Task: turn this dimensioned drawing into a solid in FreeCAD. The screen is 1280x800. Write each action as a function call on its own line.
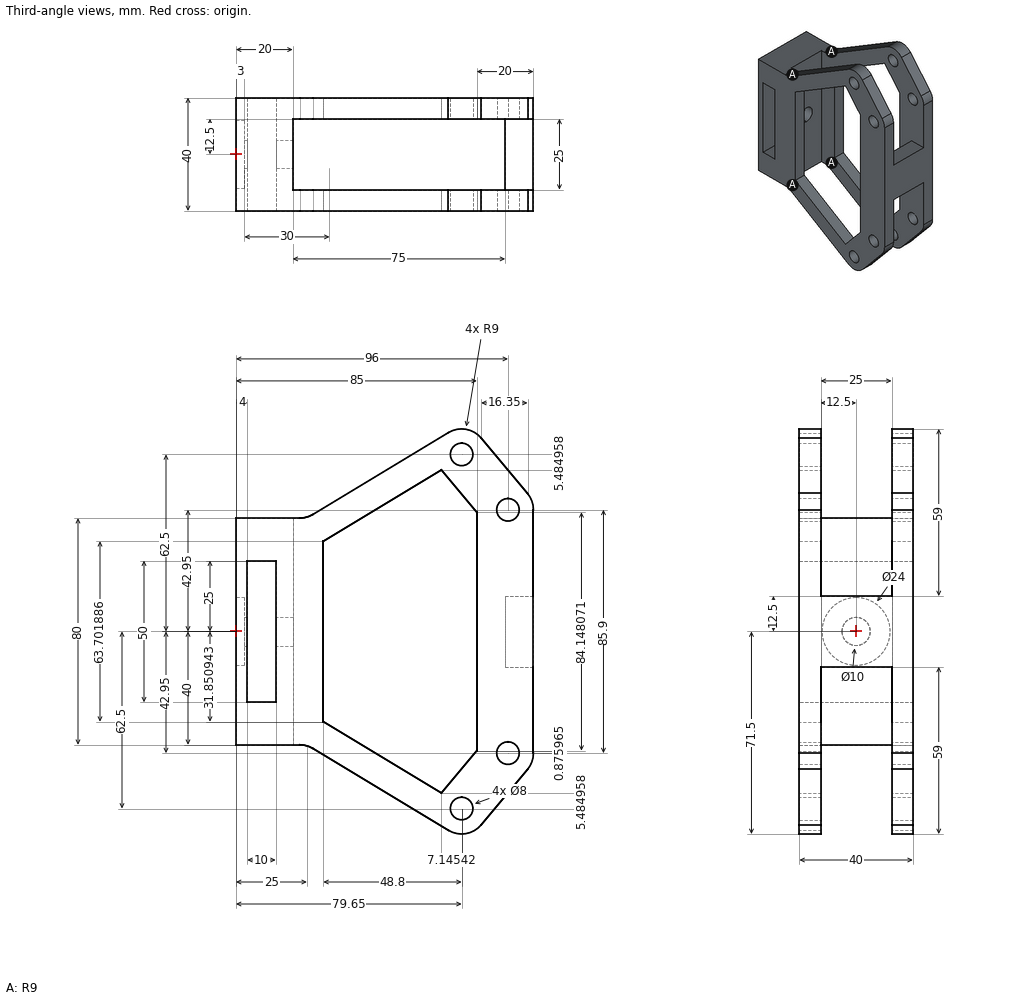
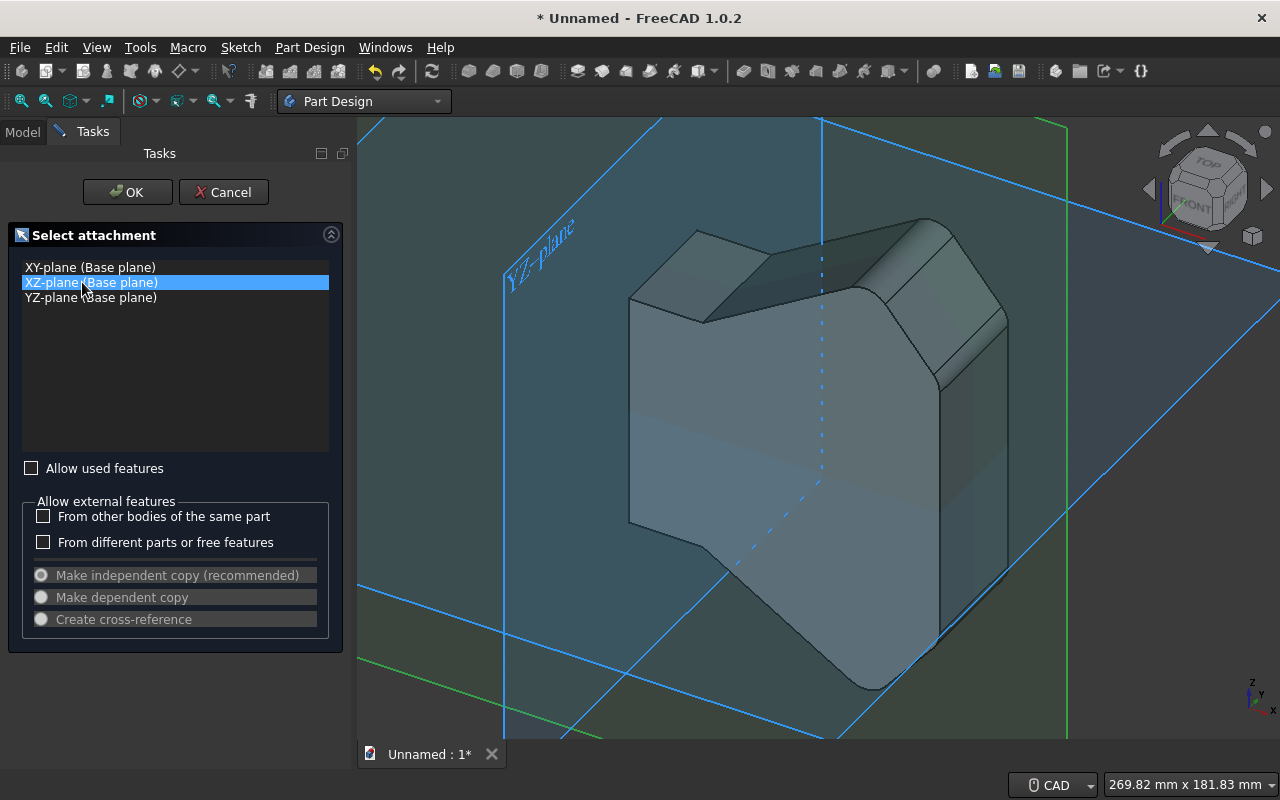
click(128, 192)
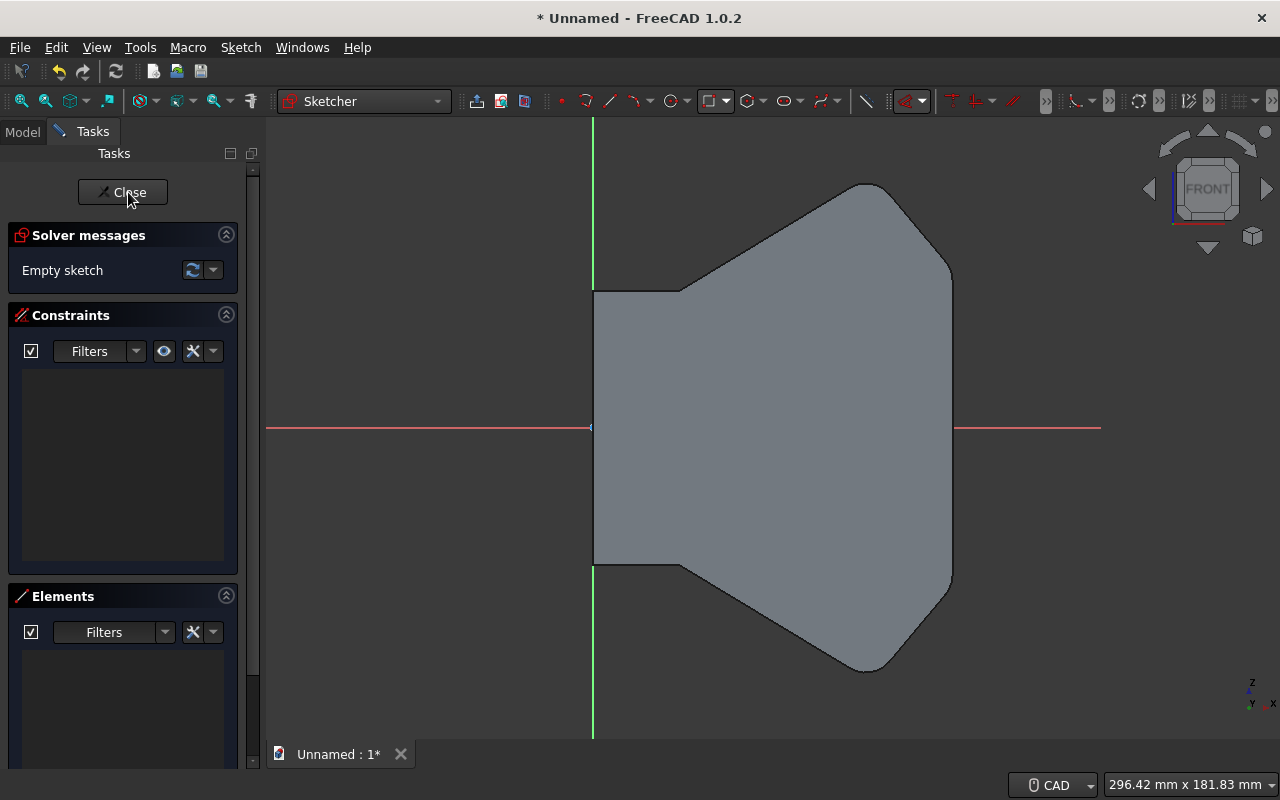
key(q)
key(s)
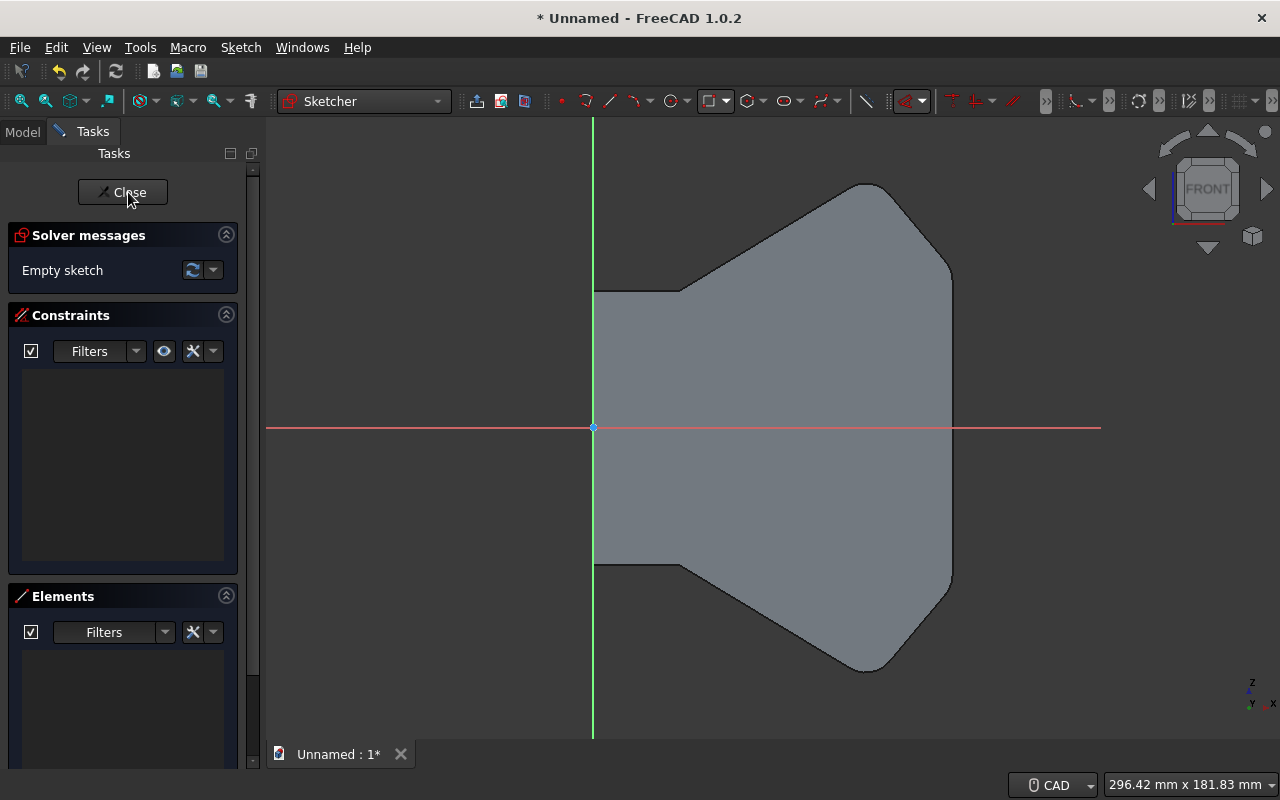
click(586, 102)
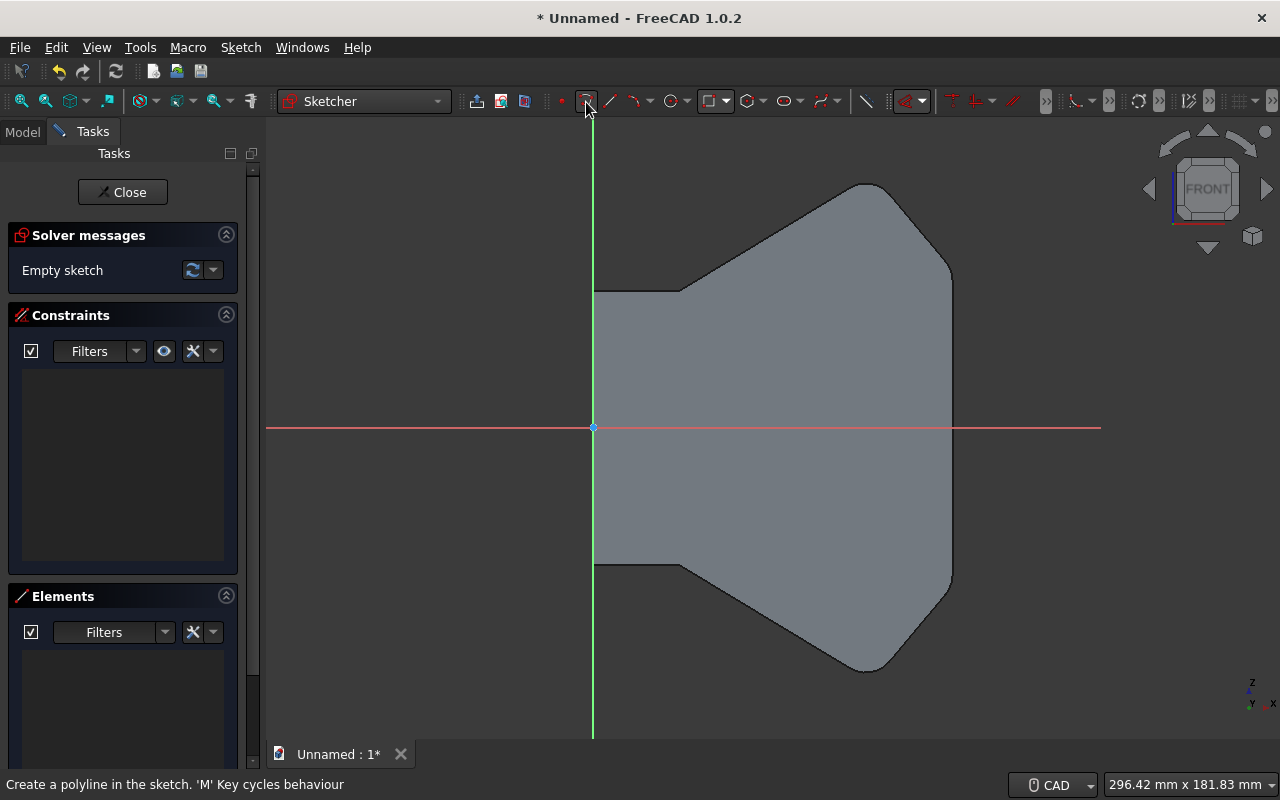
click(699, 537)
click(699, 319)
click(841, 233)
click(884, 284)
click(884, 572)
click(841, 623)
click(699, 538)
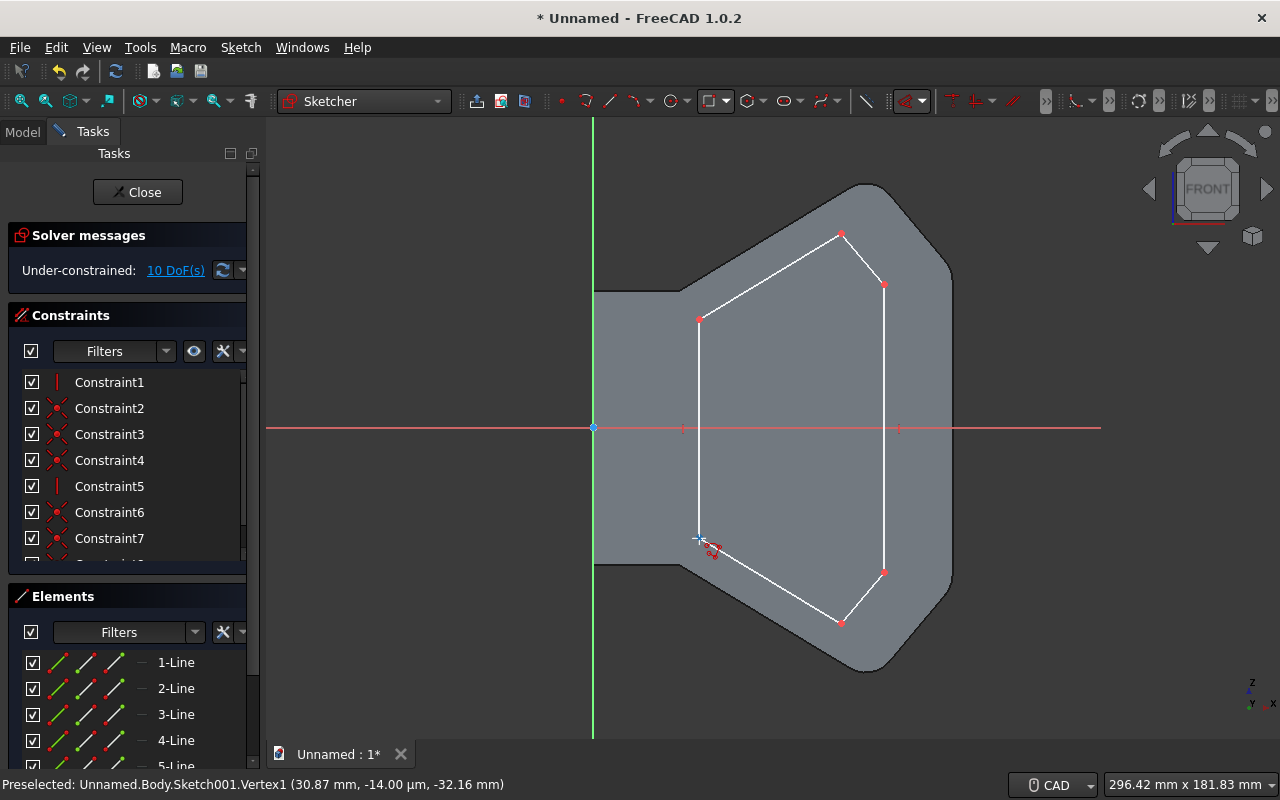
key(g)
key(r)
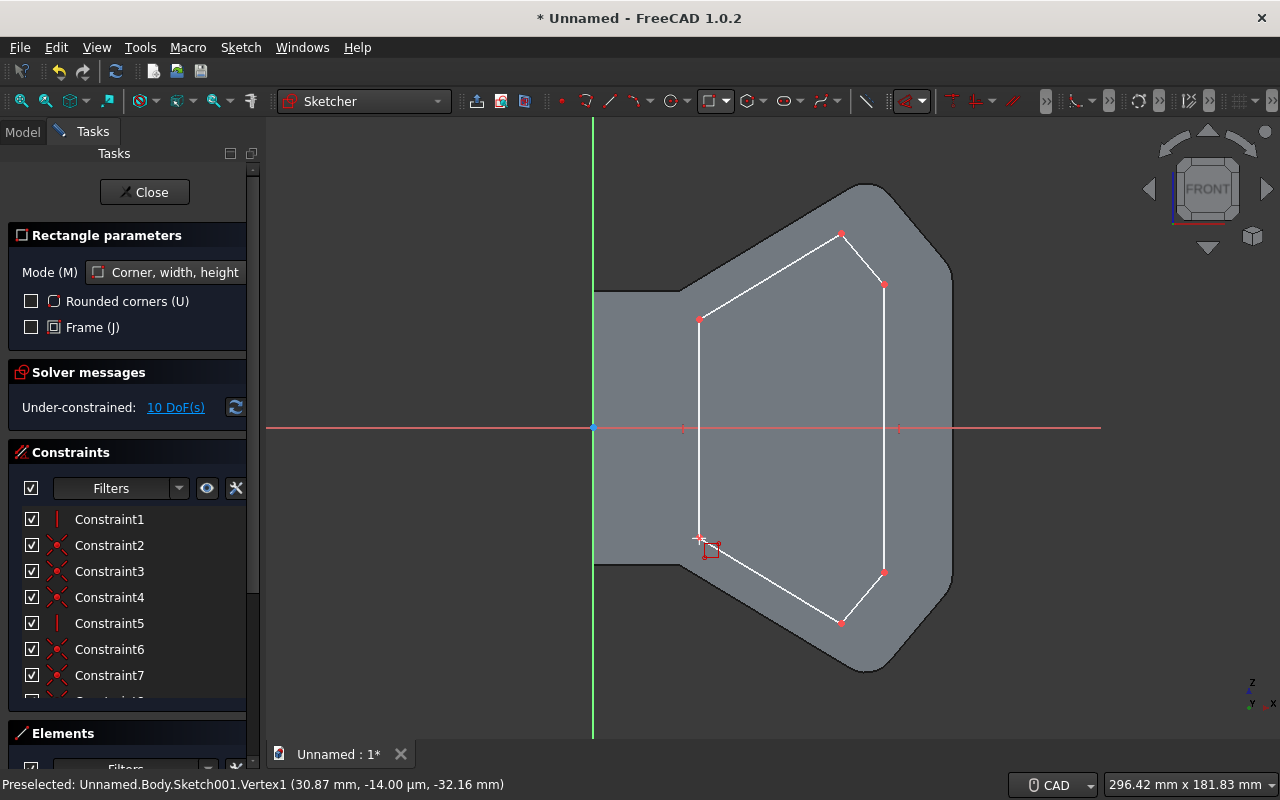
click(607, 342)
move(641, 514)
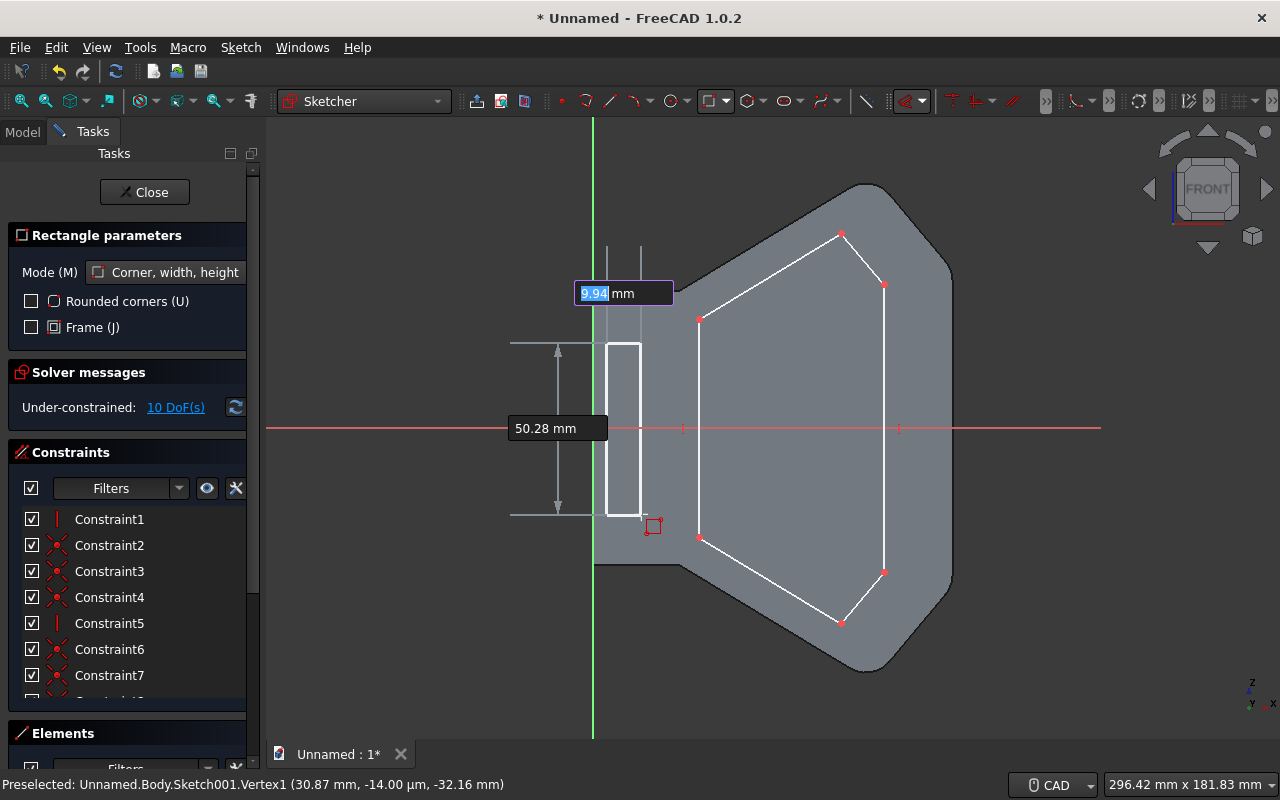
text(10)
key(Tab)
text(50)
key(Return)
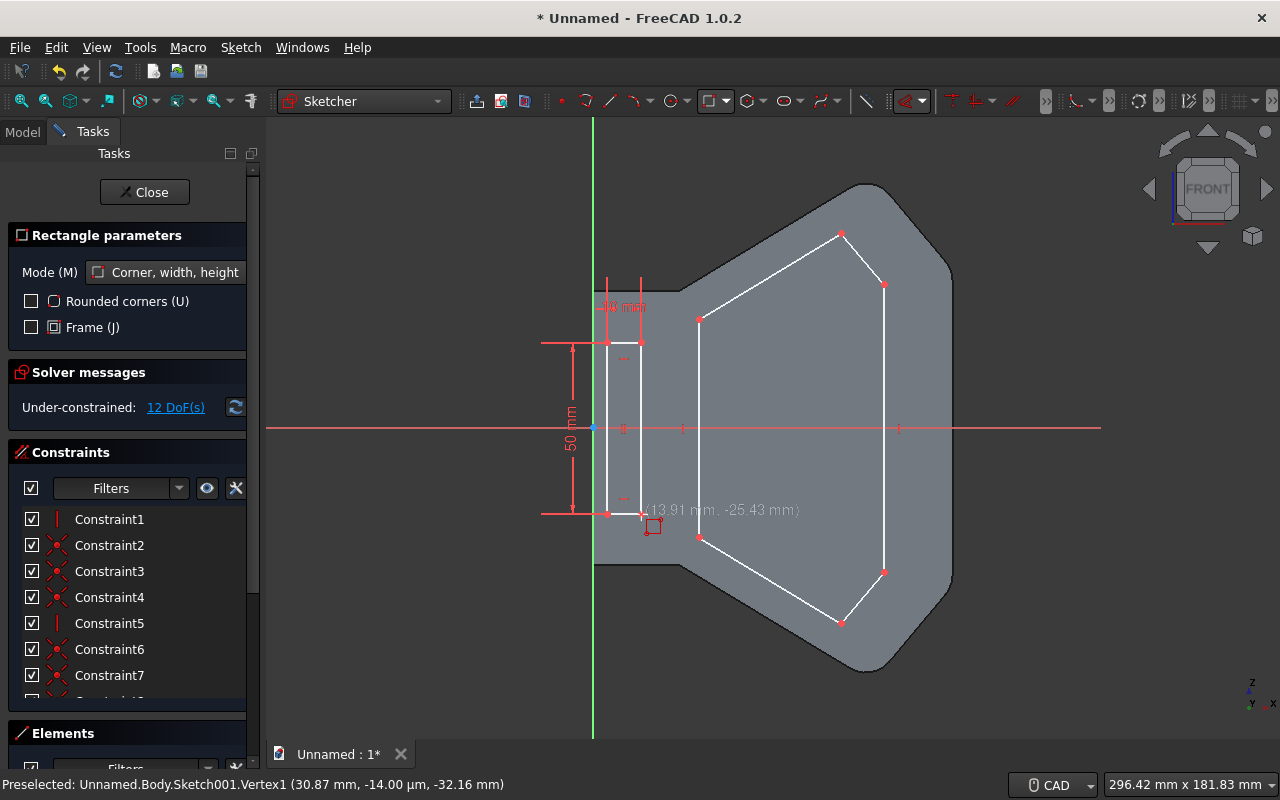
key(g)
key(c)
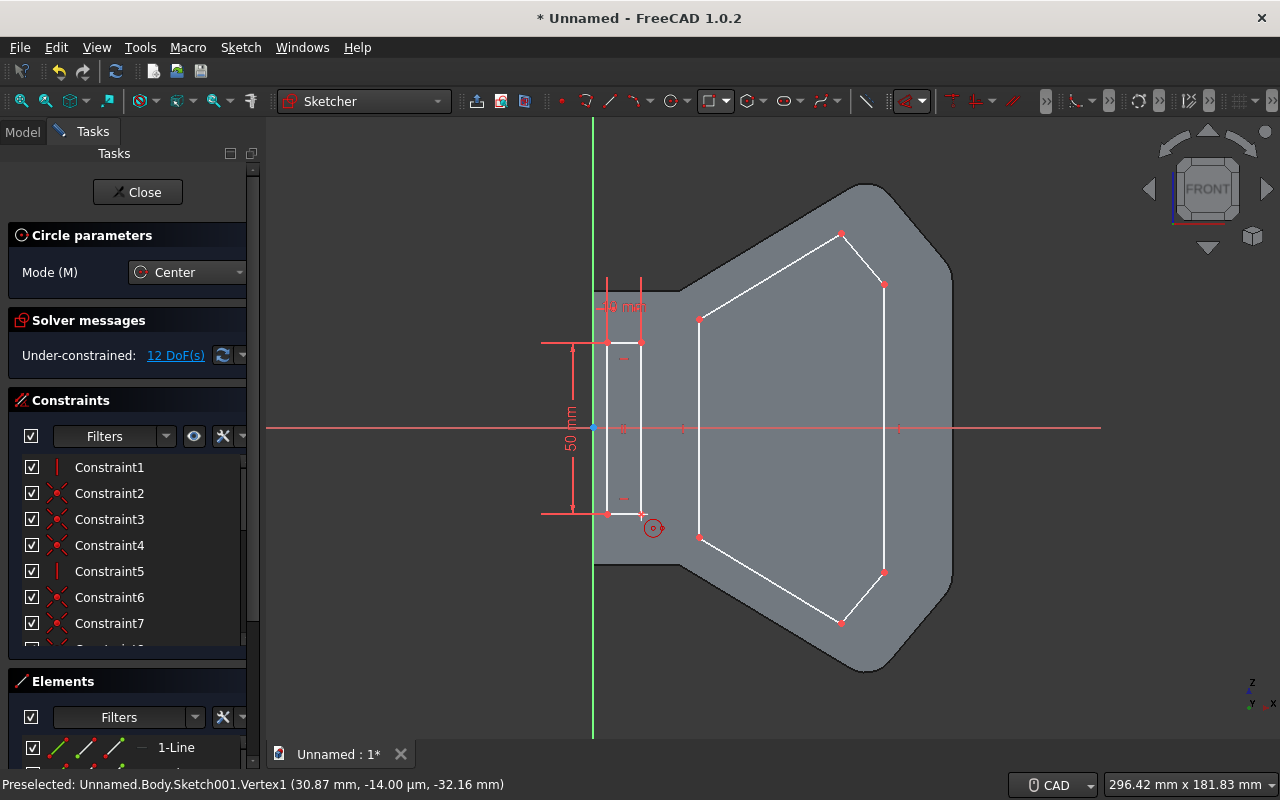
scroll(866, 642, up, 3)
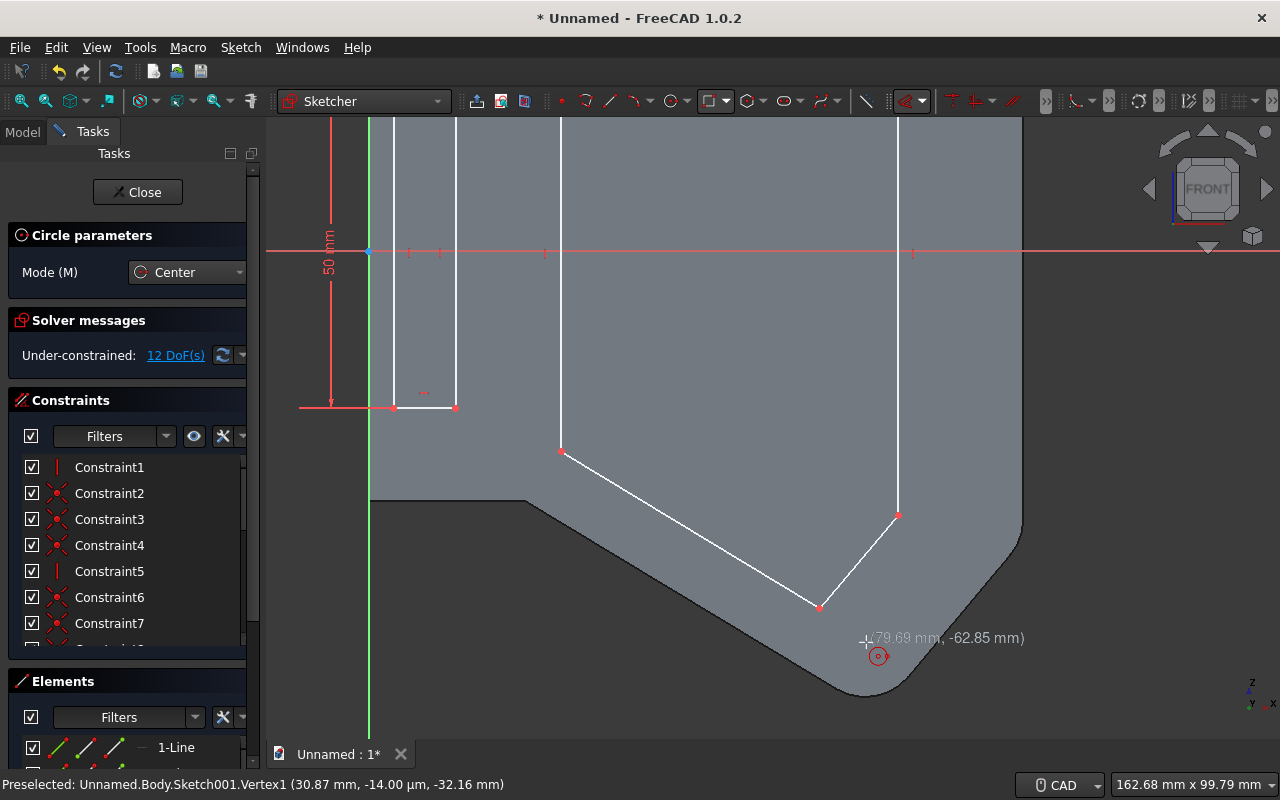
click(865, 641)
move(883, 623)